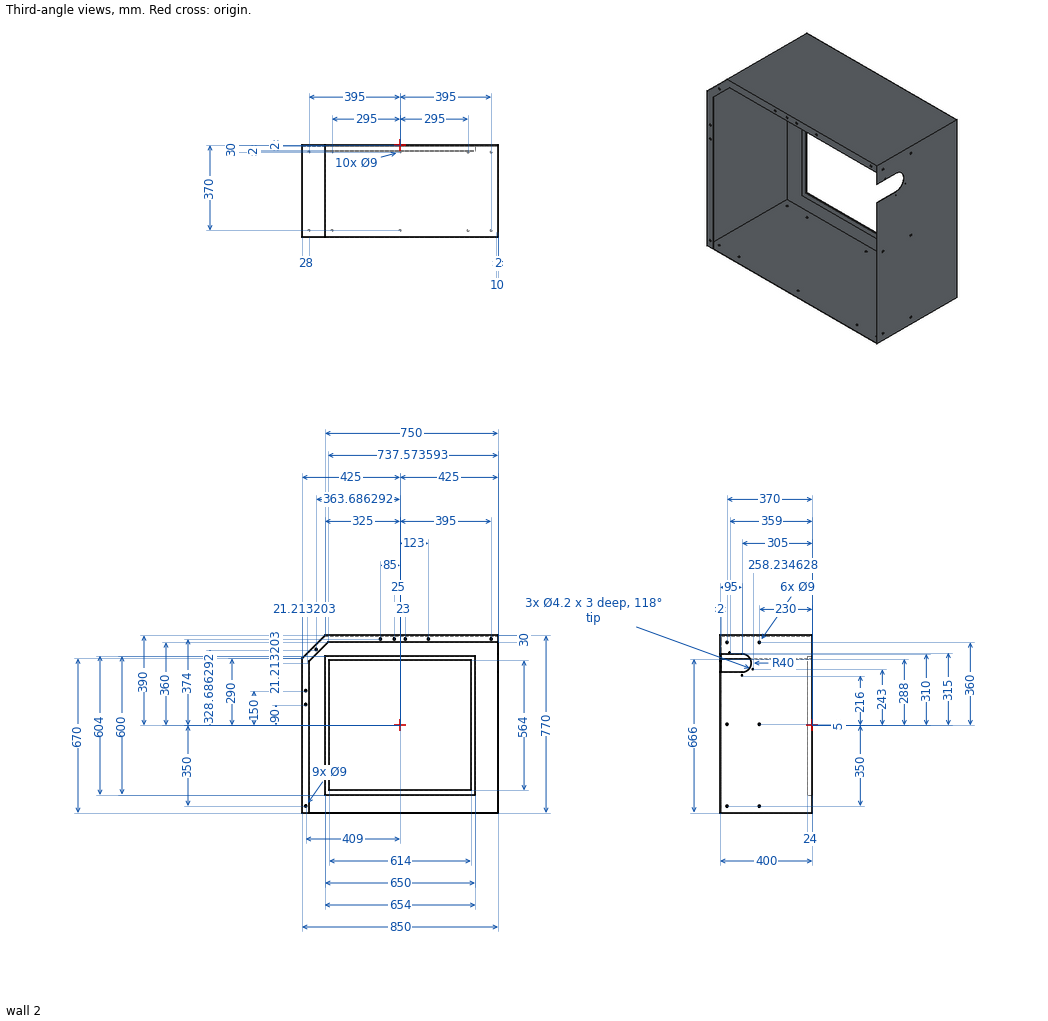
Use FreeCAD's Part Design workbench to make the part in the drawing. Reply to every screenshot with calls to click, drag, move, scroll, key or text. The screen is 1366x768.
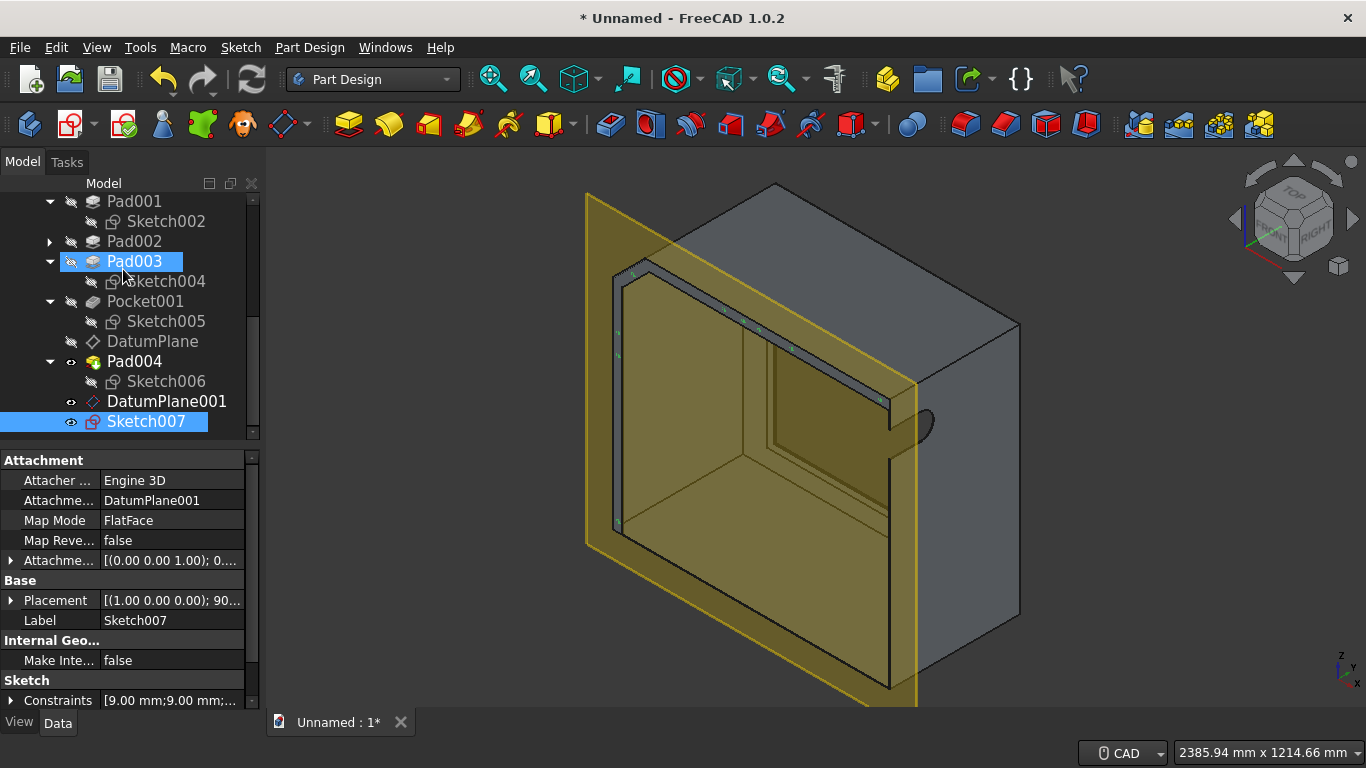
click(612, 124)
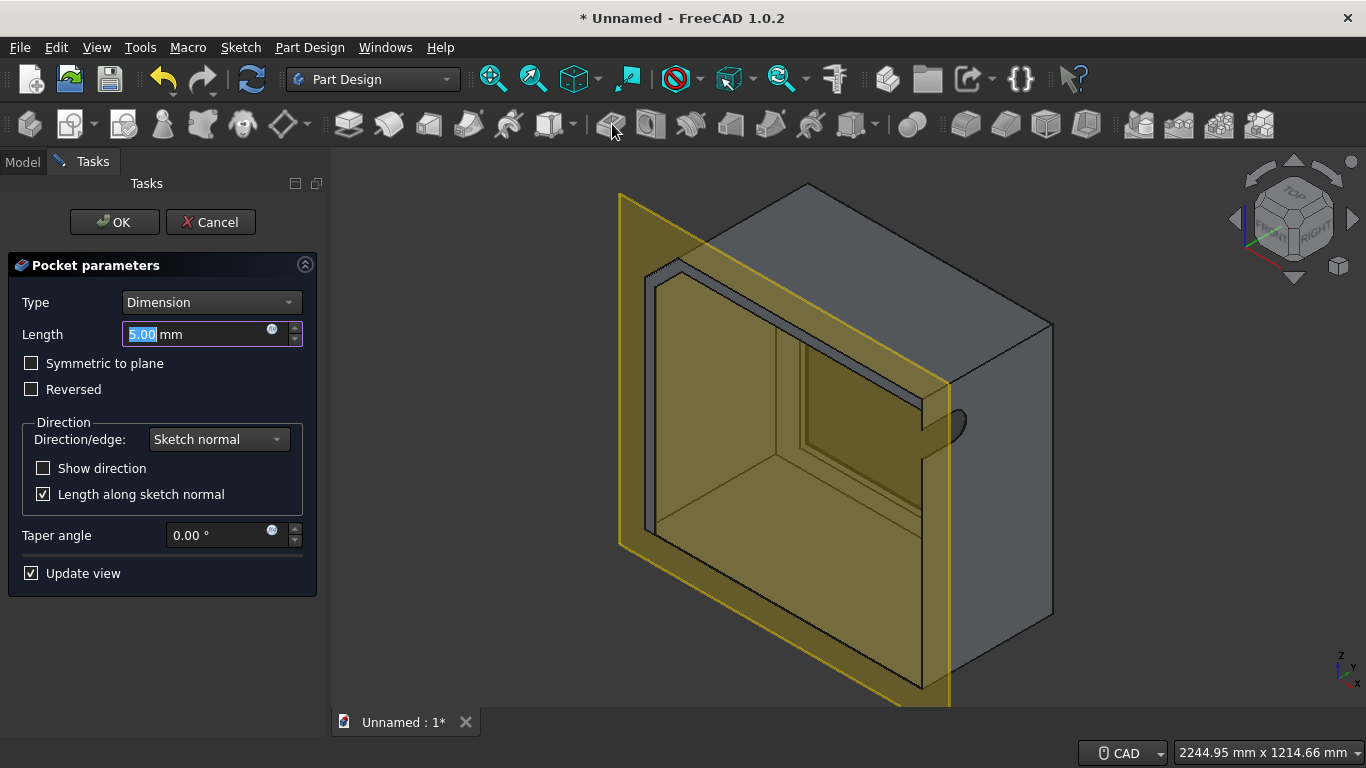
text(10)
key(Tab)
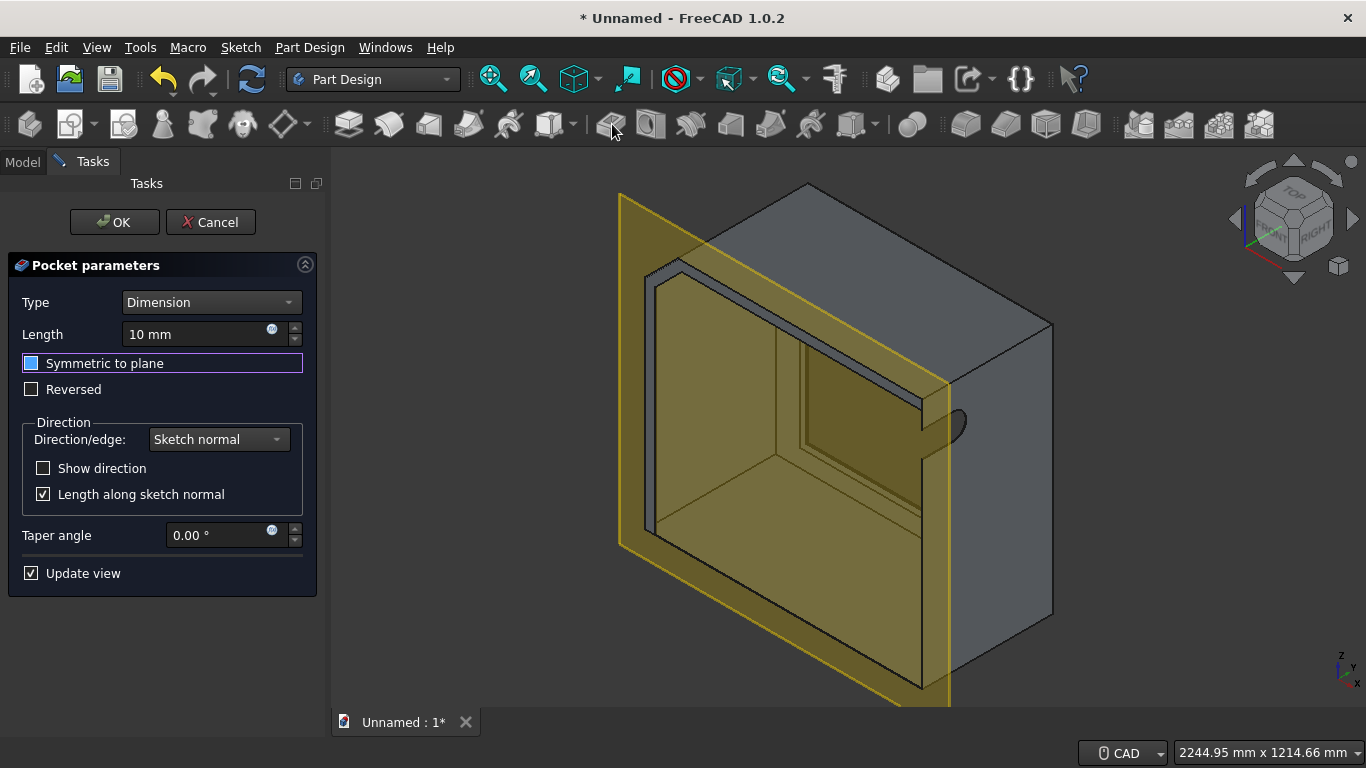
click(30, 389)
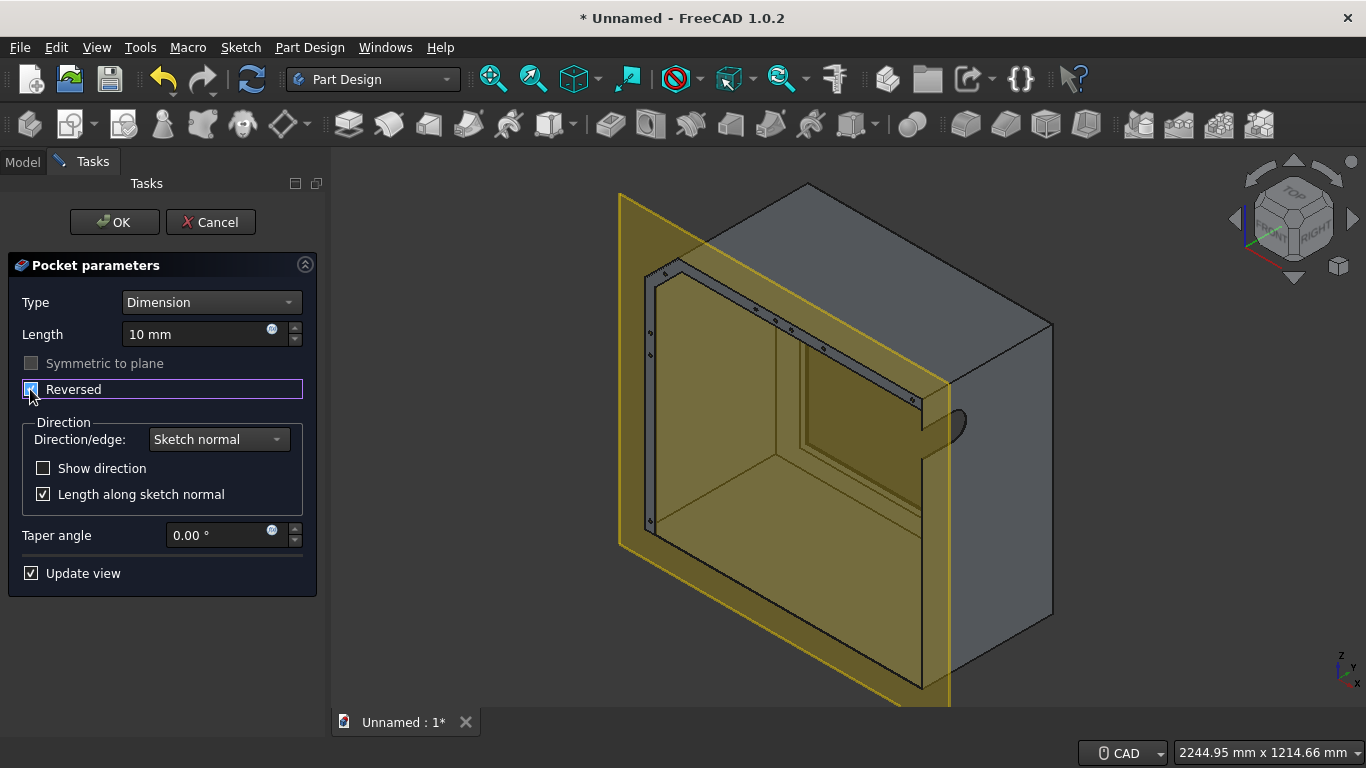
click(115, 222)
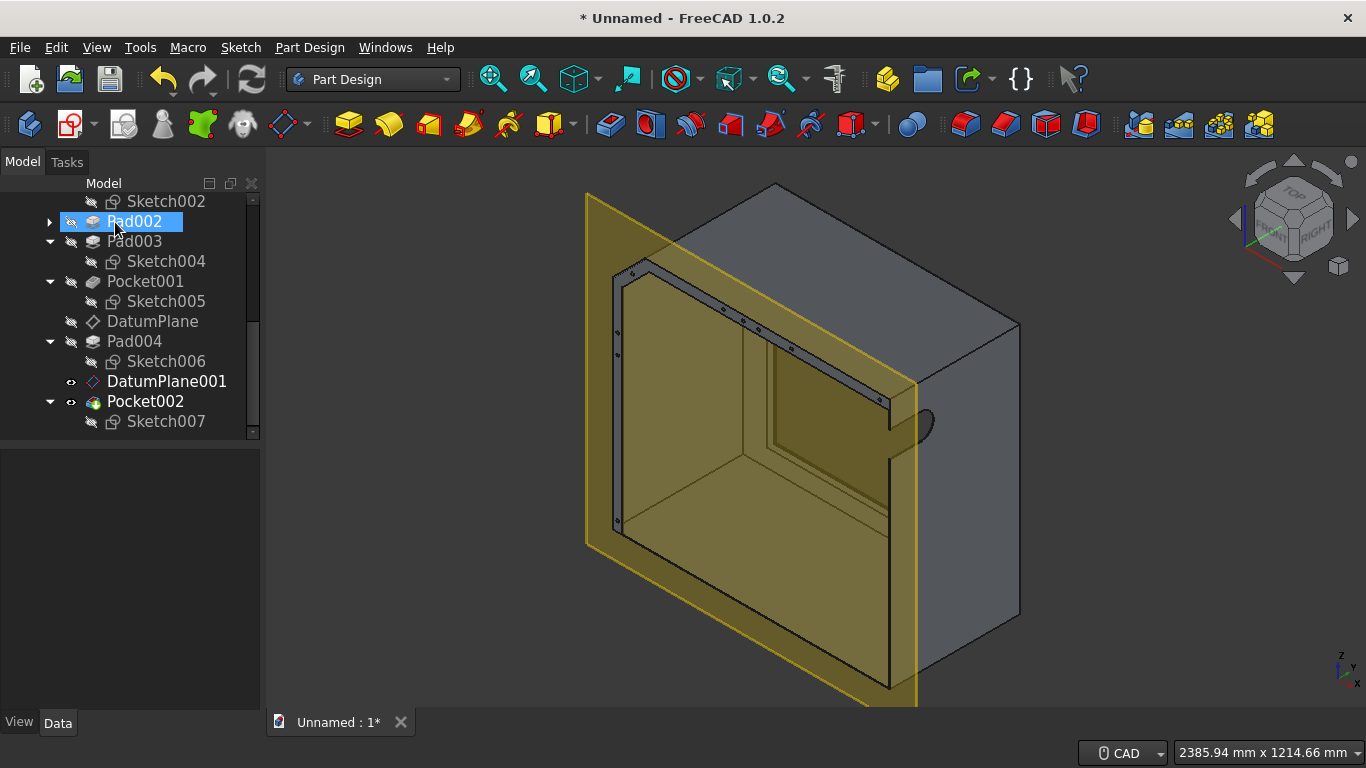
click(116, 382)
key(space)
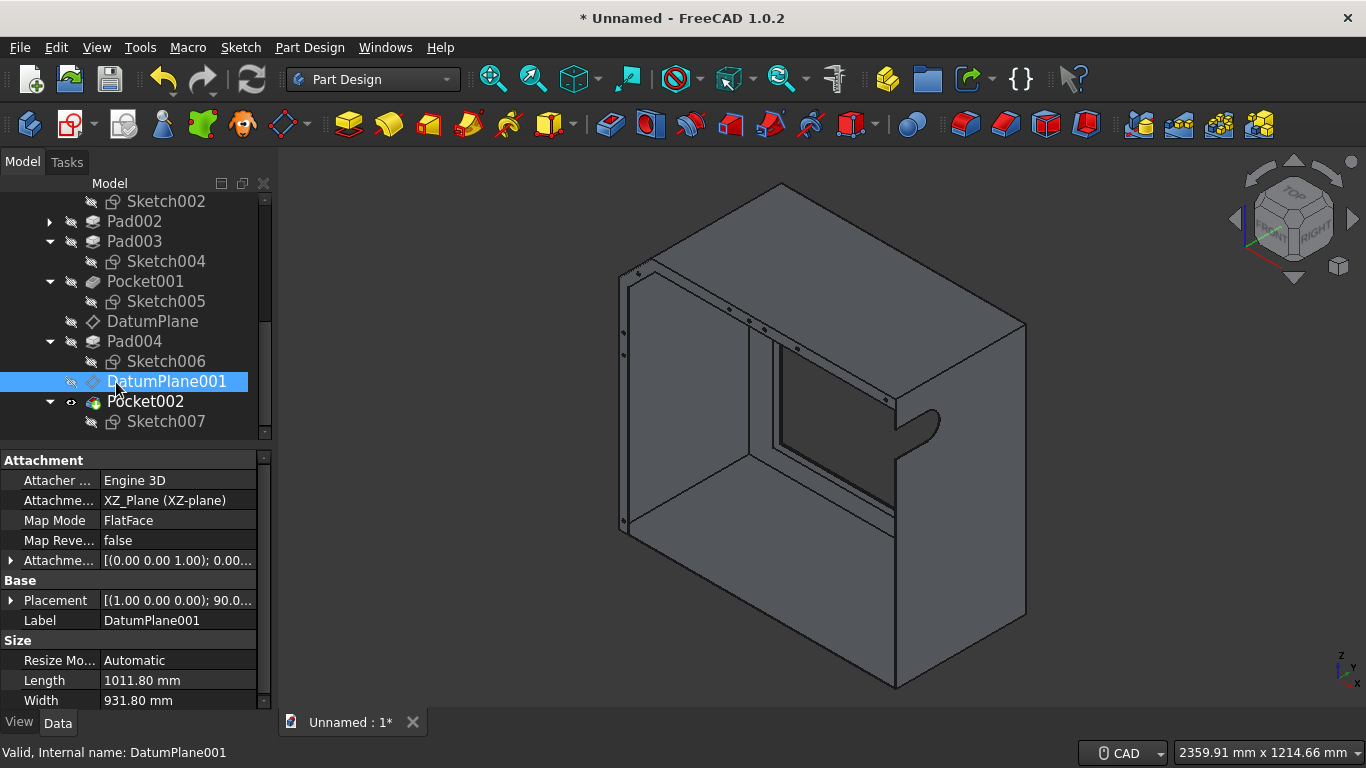
scroll(160, 317, down, 3)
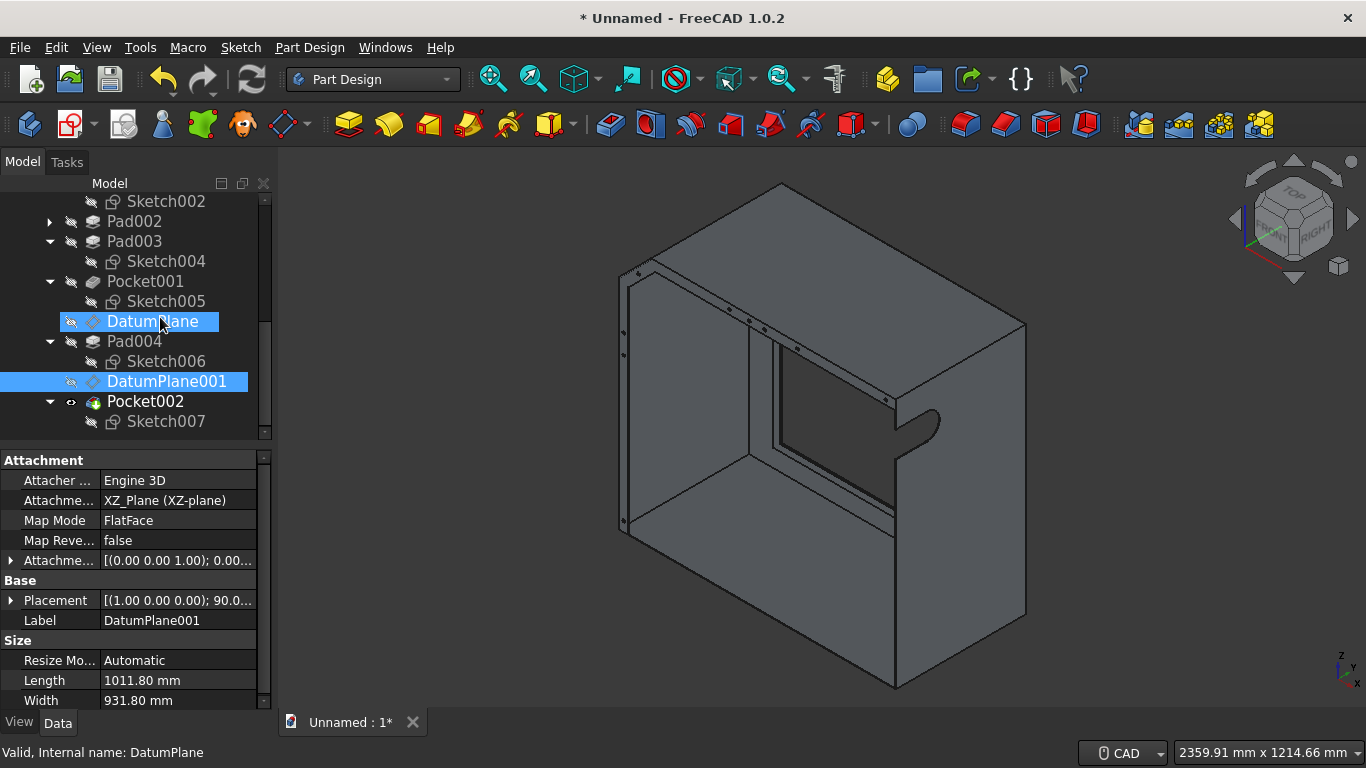
scroll(160, 317, up, 15)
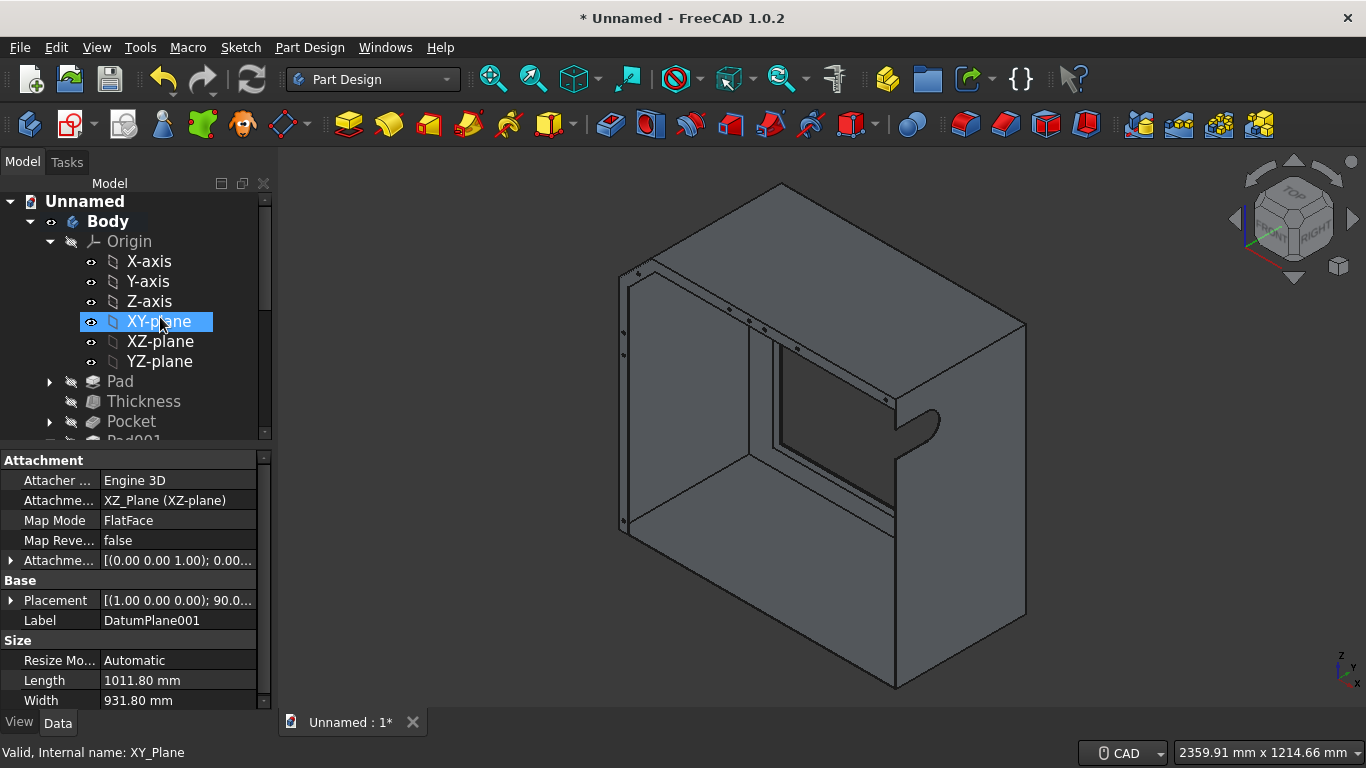
click(136, 322)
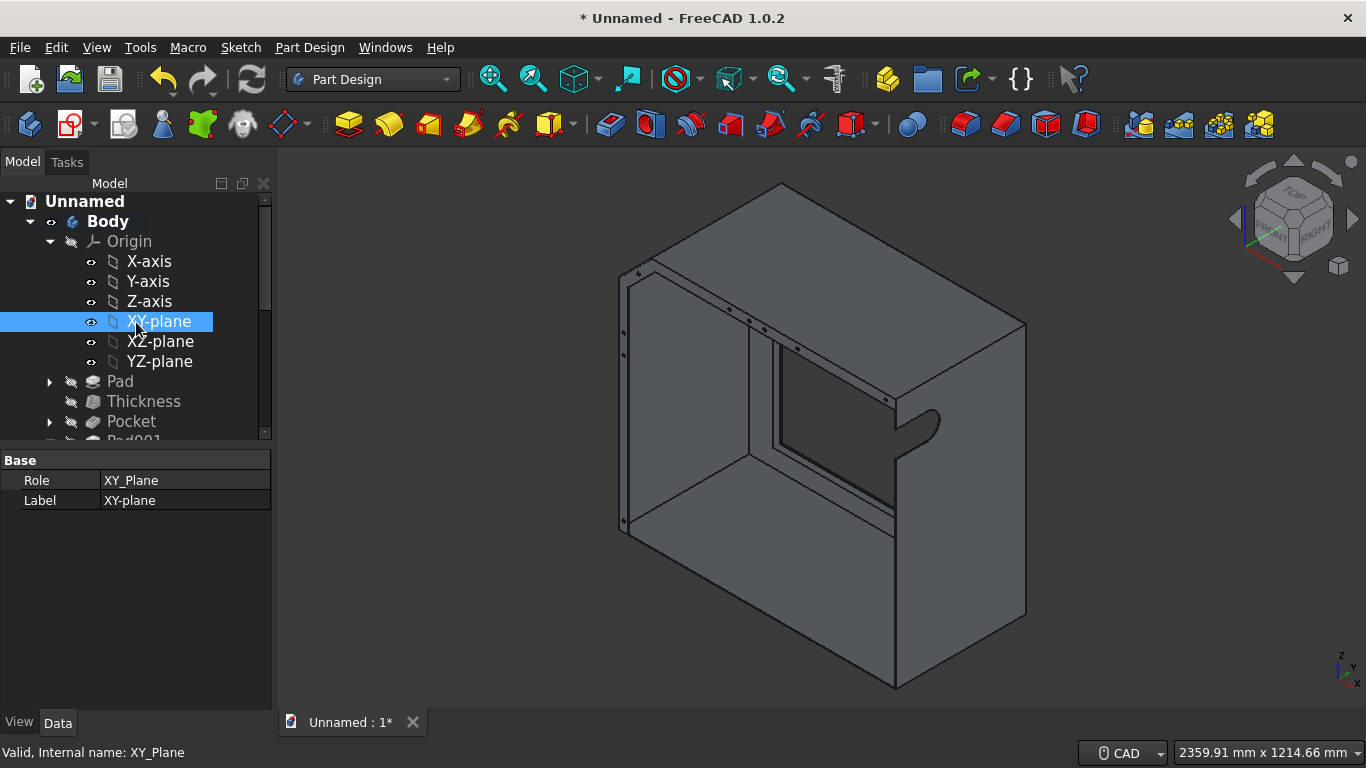
click(284, 124)